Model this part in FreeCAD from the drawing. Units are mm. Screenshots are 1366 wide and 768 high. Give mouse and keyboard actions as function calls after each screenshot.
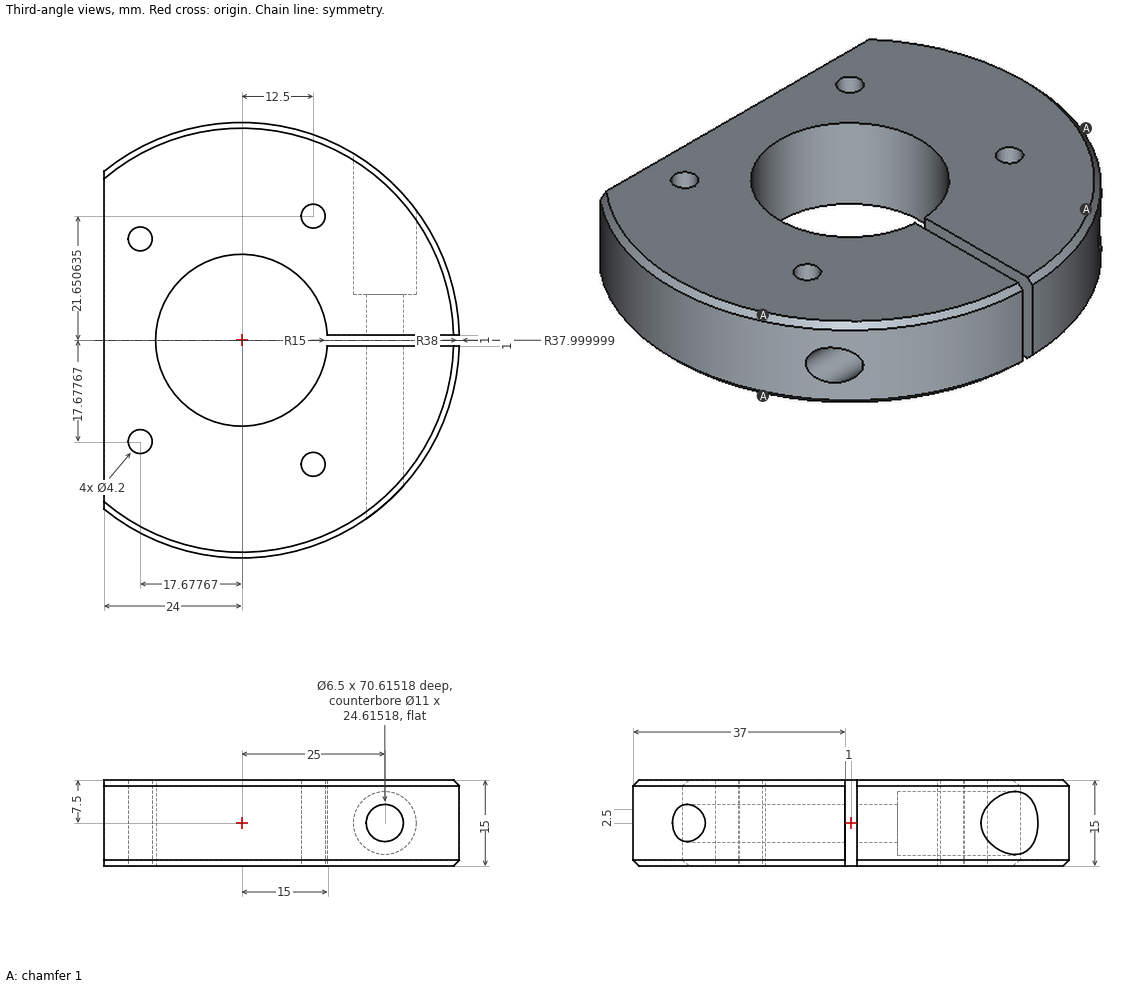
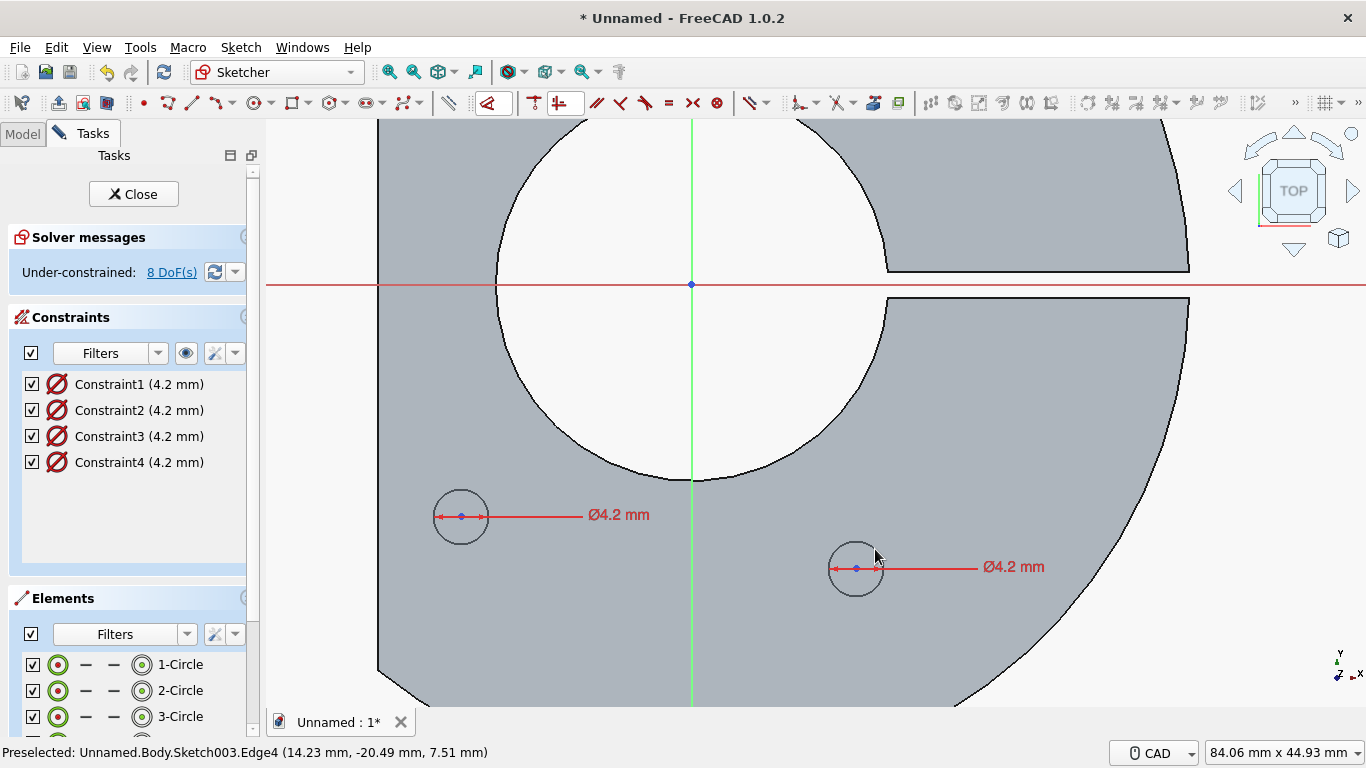
click(461, 517)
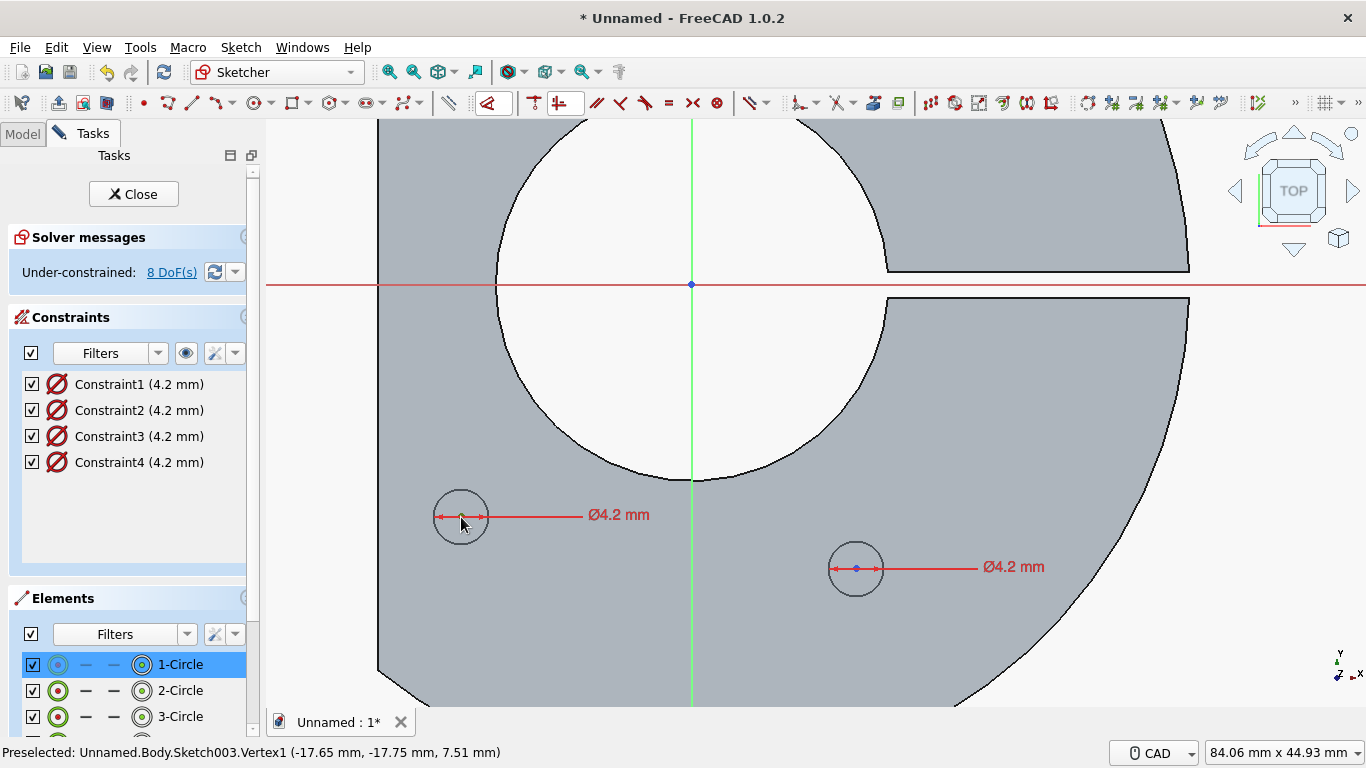
scroll(856, 569, down, 3)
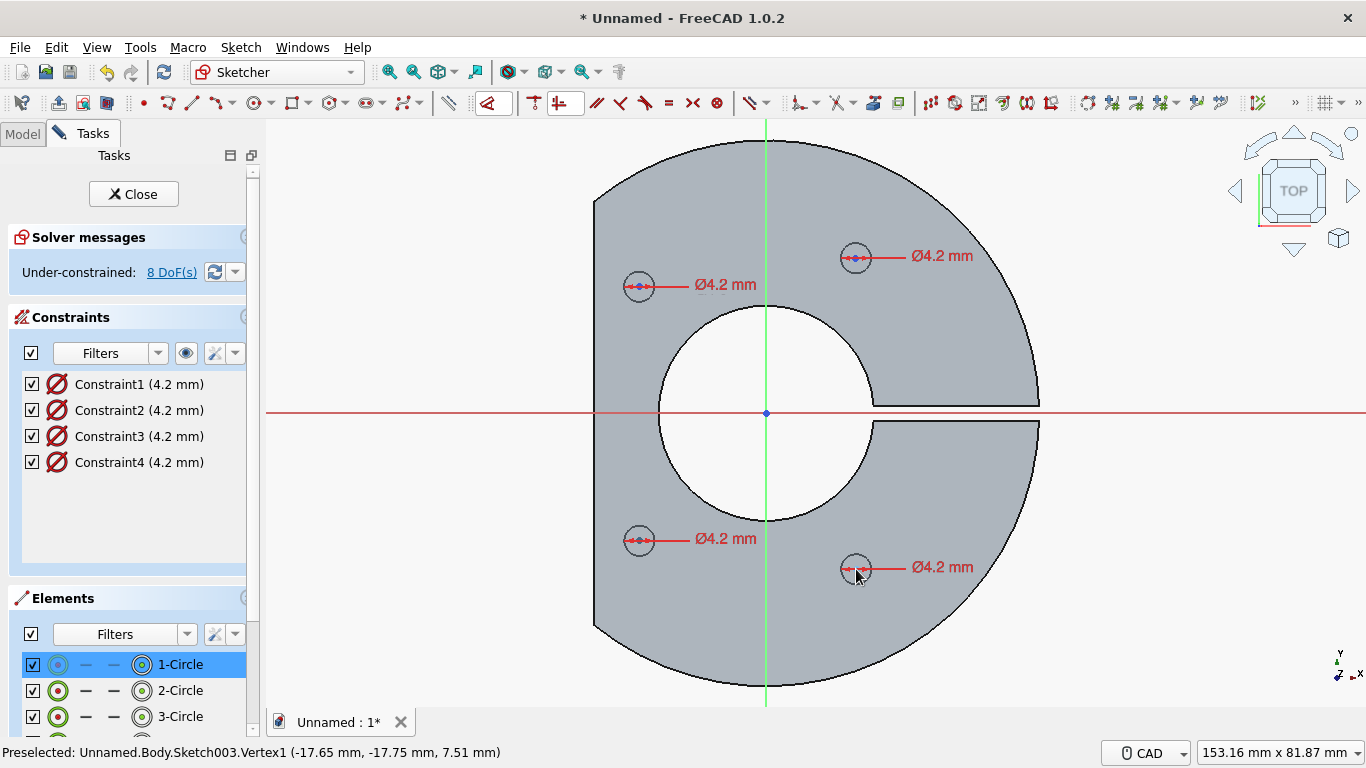
click(639, 287)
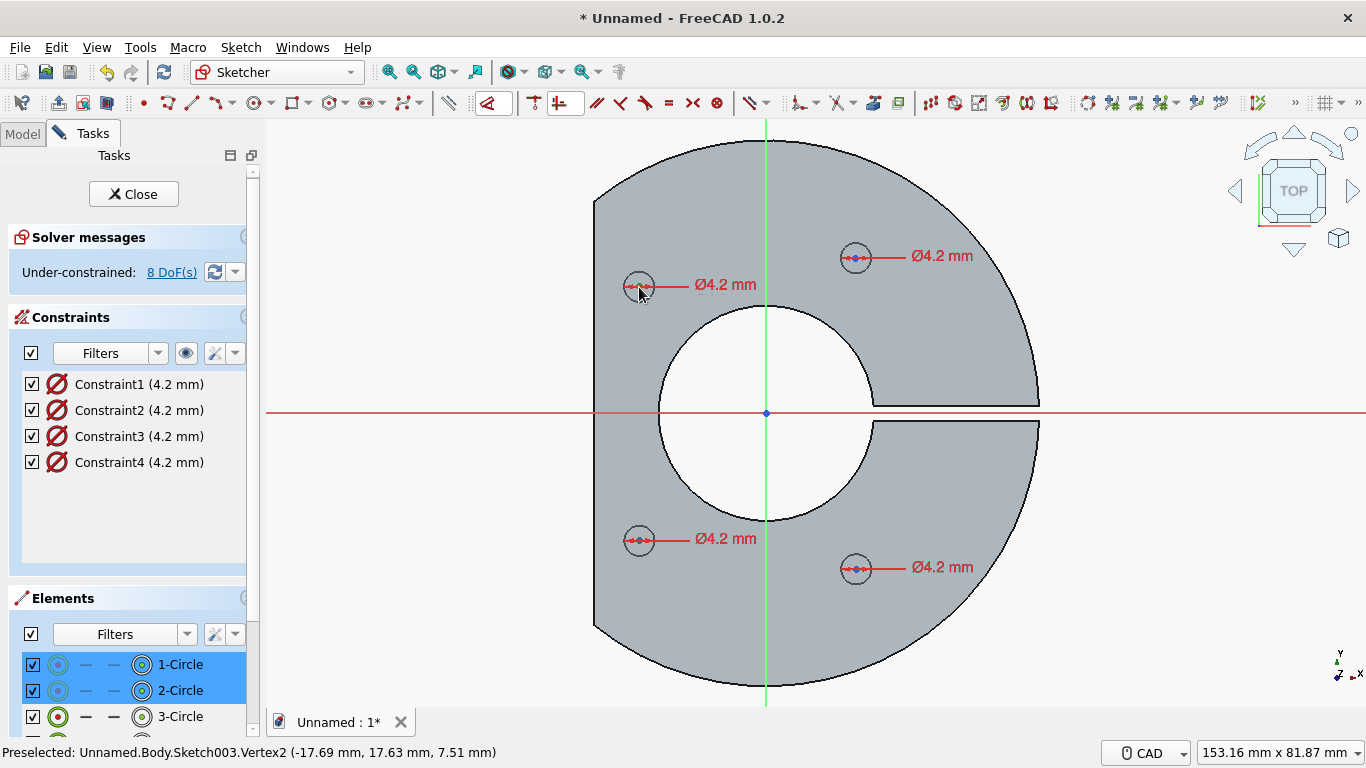
click(359, 413)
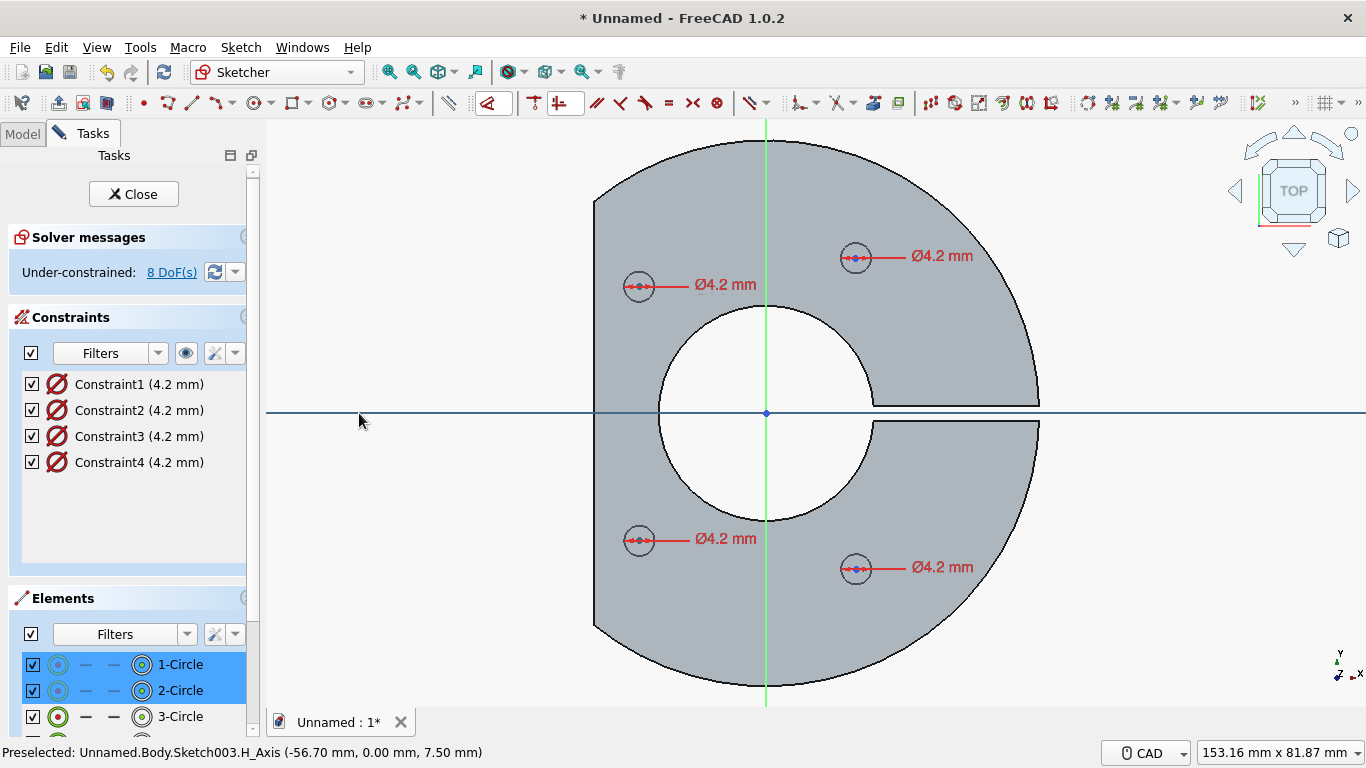
click(694, 104)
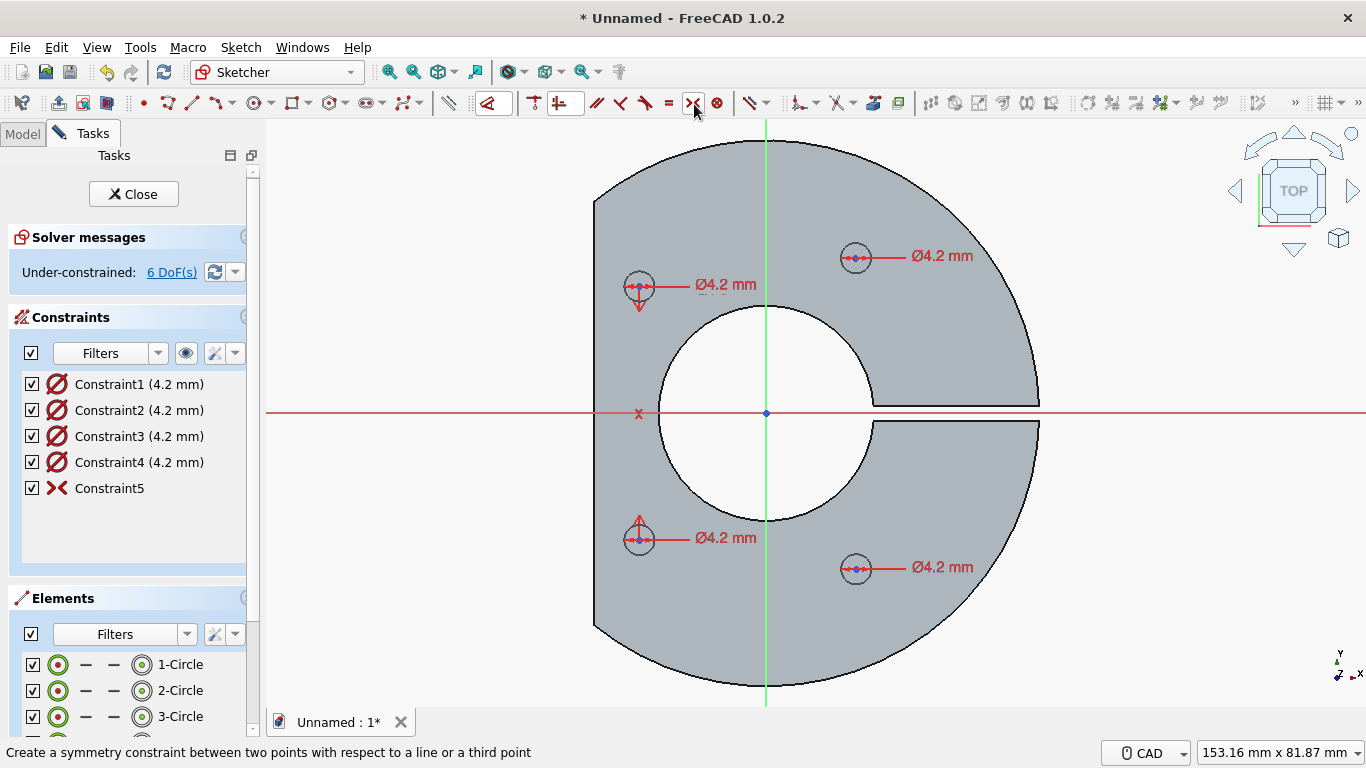
click(856, 258)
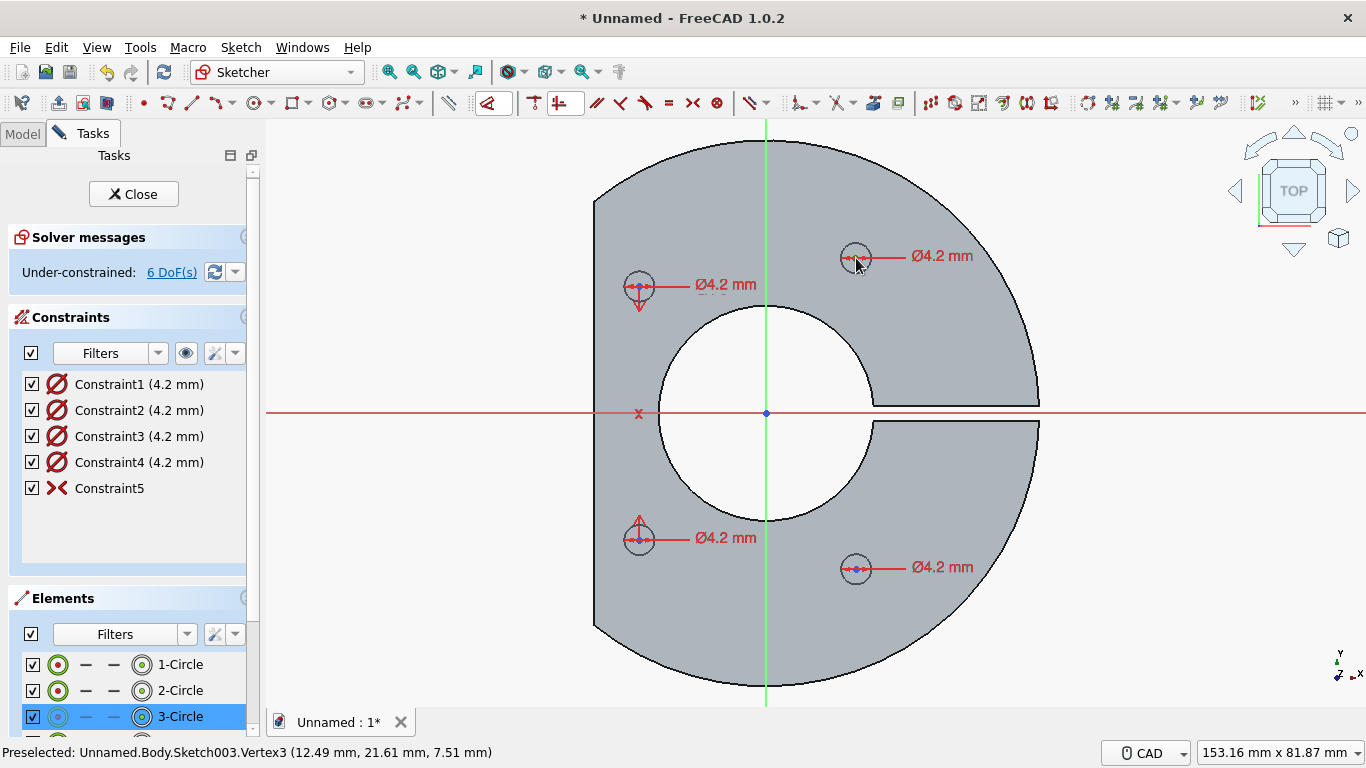
click(856, 569)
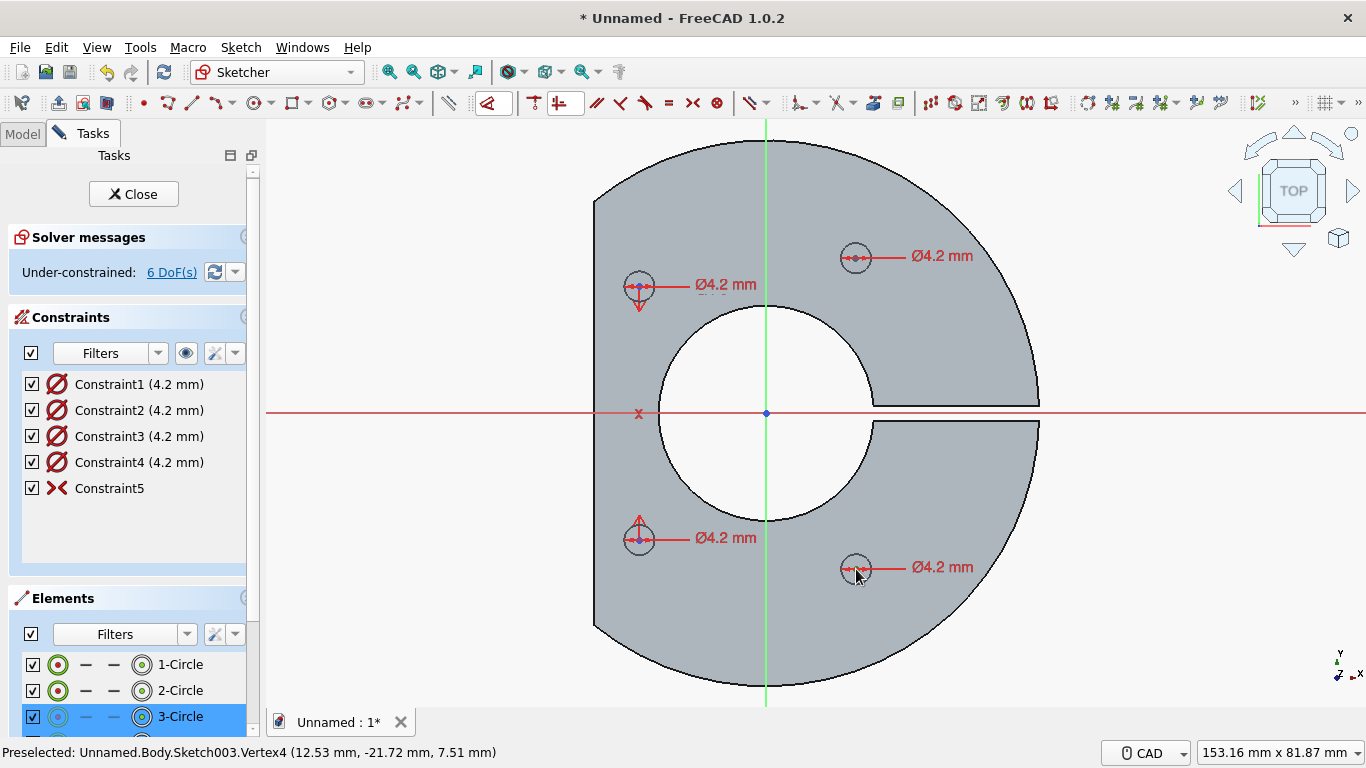
click(359, 413)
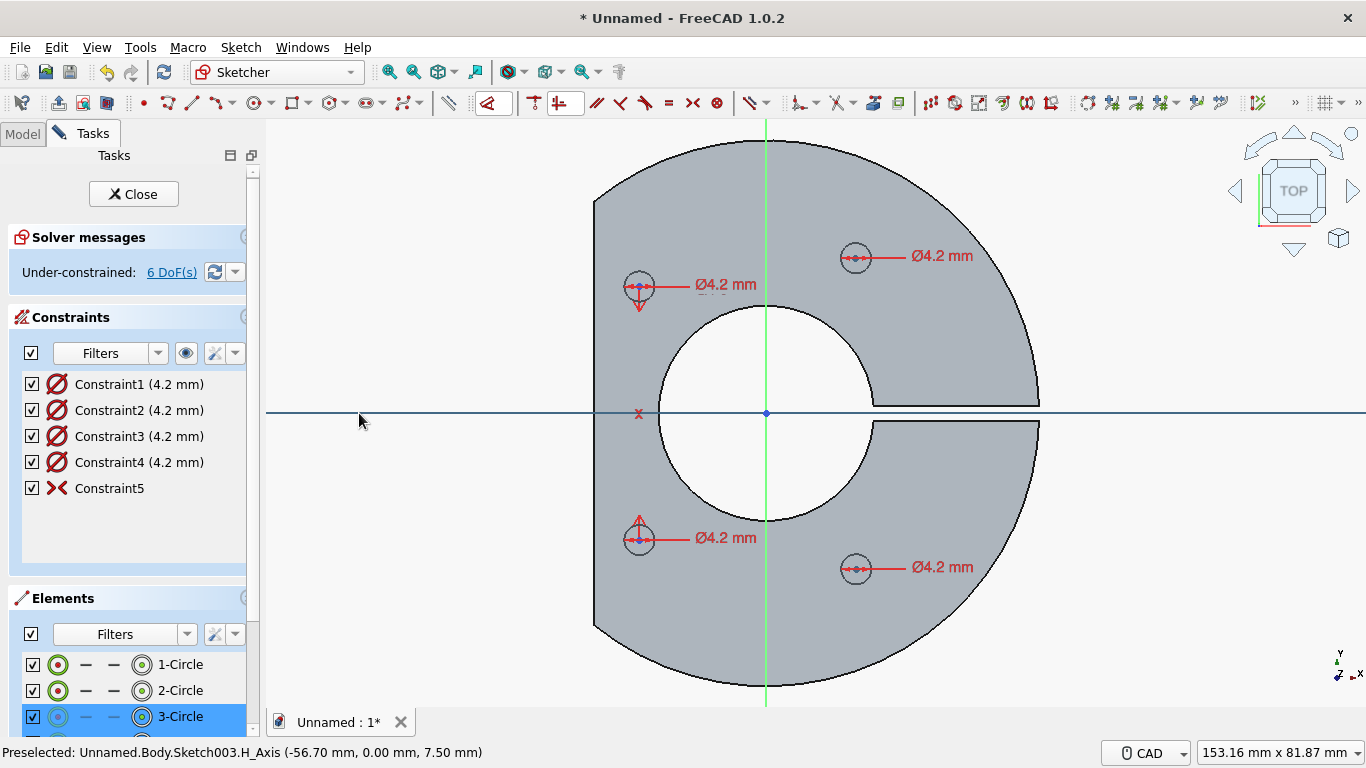
click(694, 104)